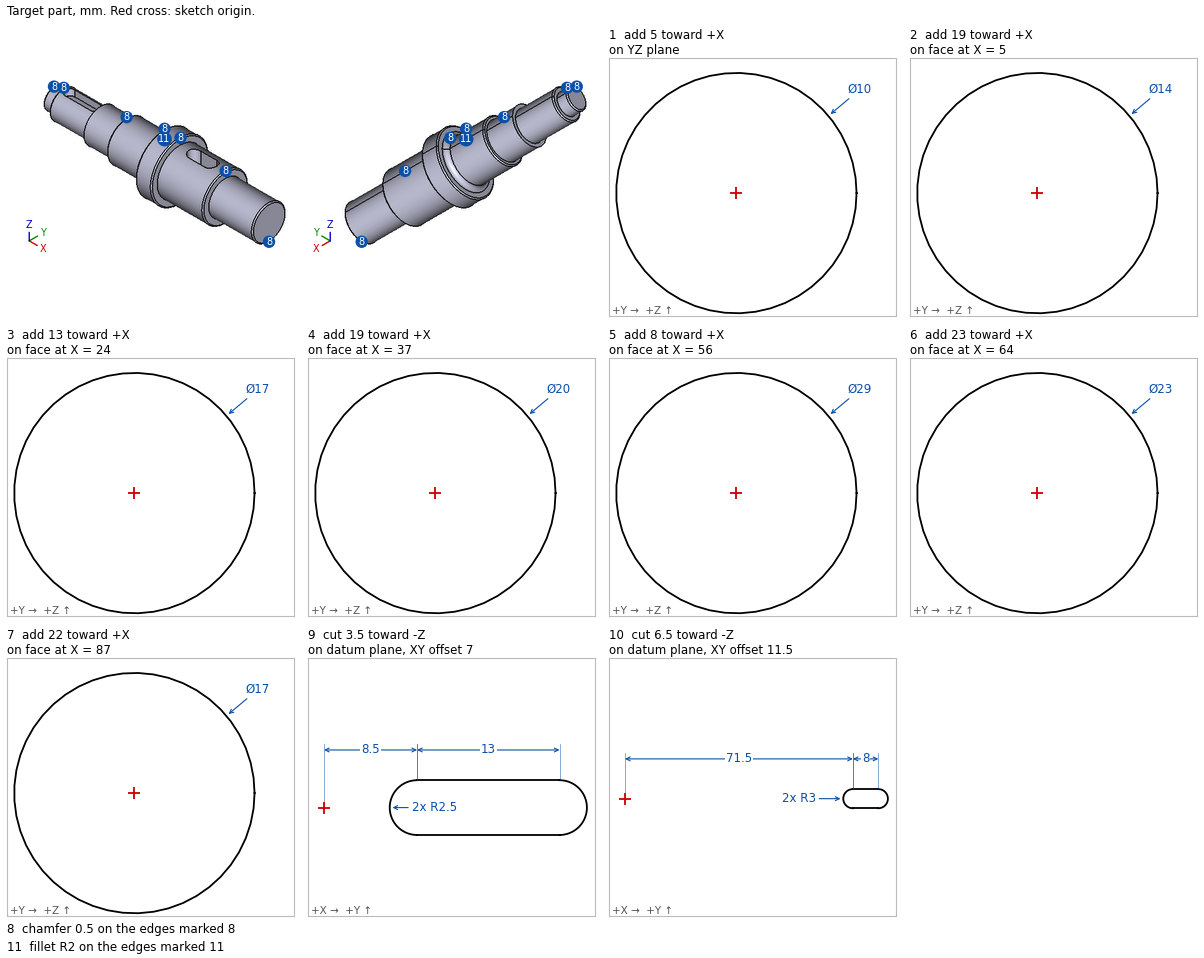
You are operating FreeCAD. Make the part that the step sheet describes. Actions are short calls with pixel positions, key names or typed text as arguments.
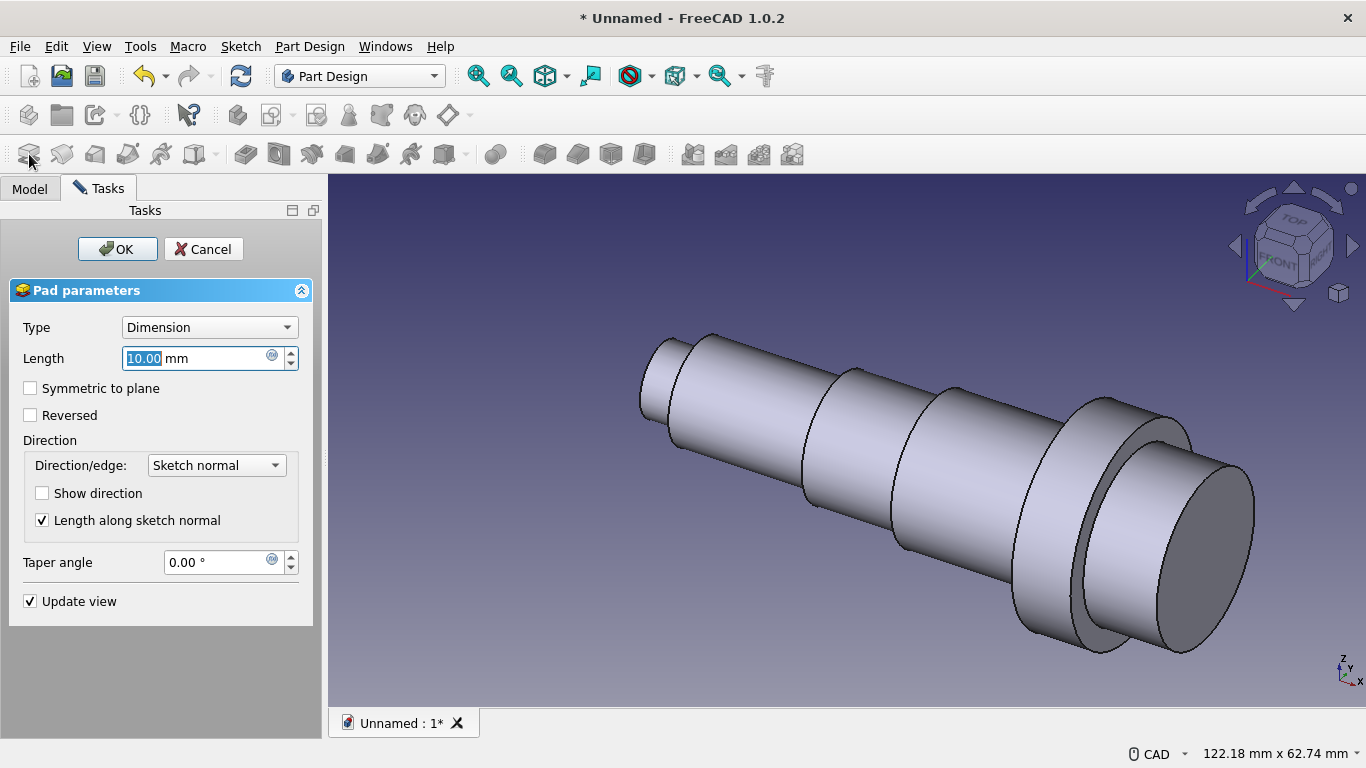
text(23)
key(Tab)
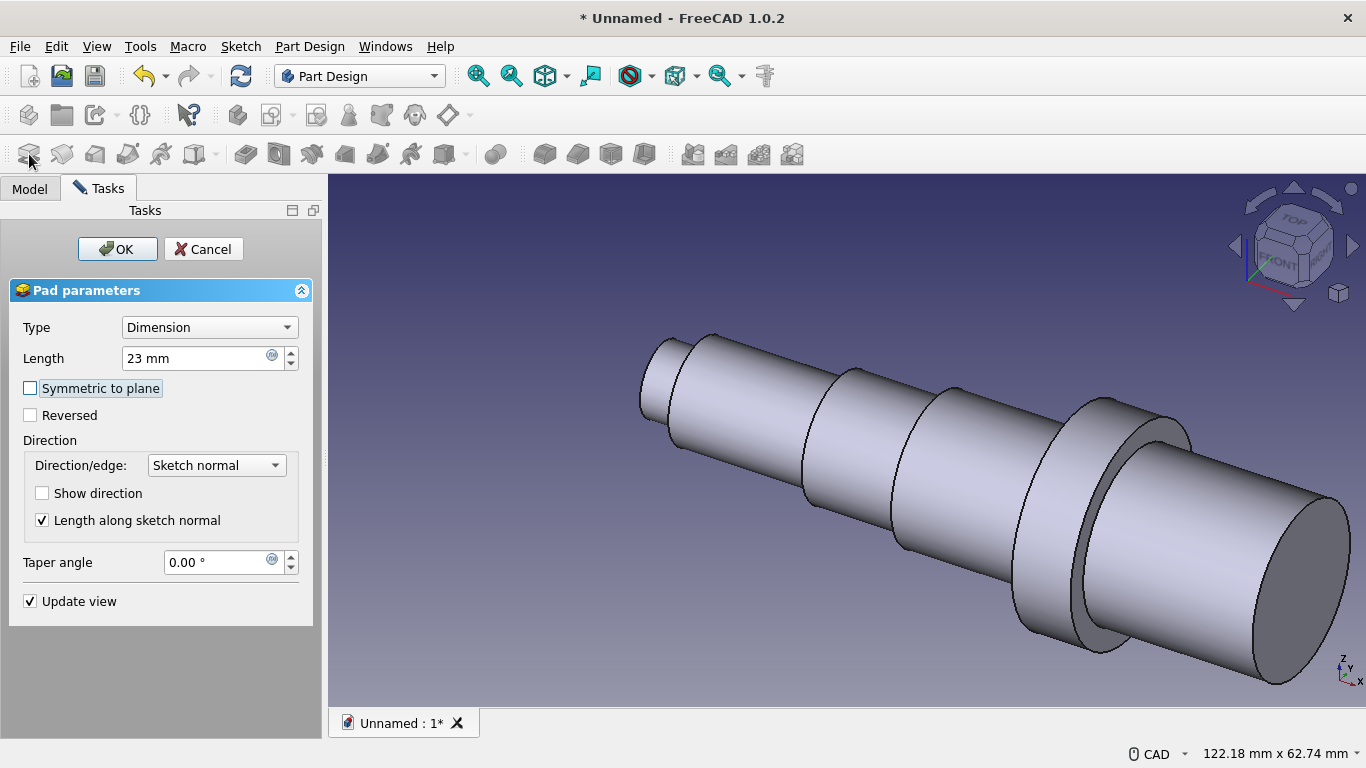
click(118, 249)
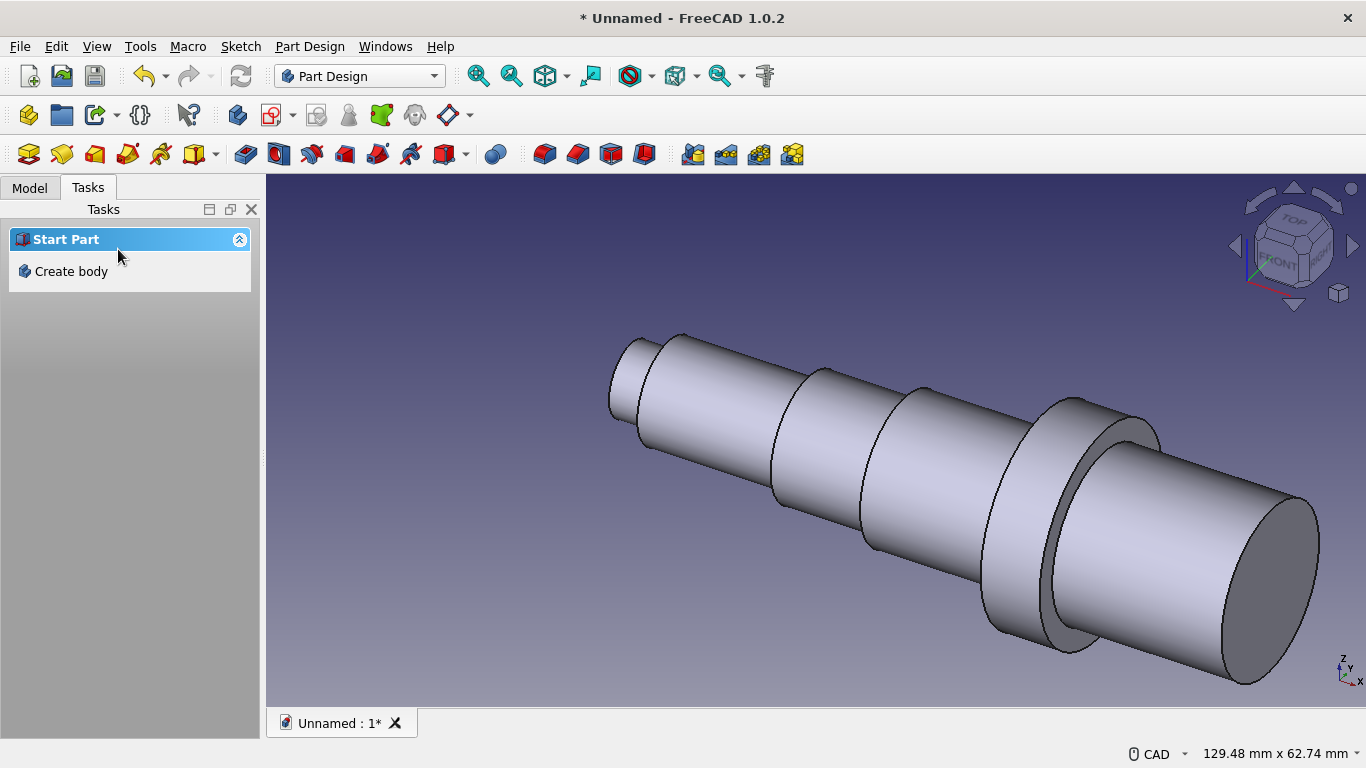
click(479, 76)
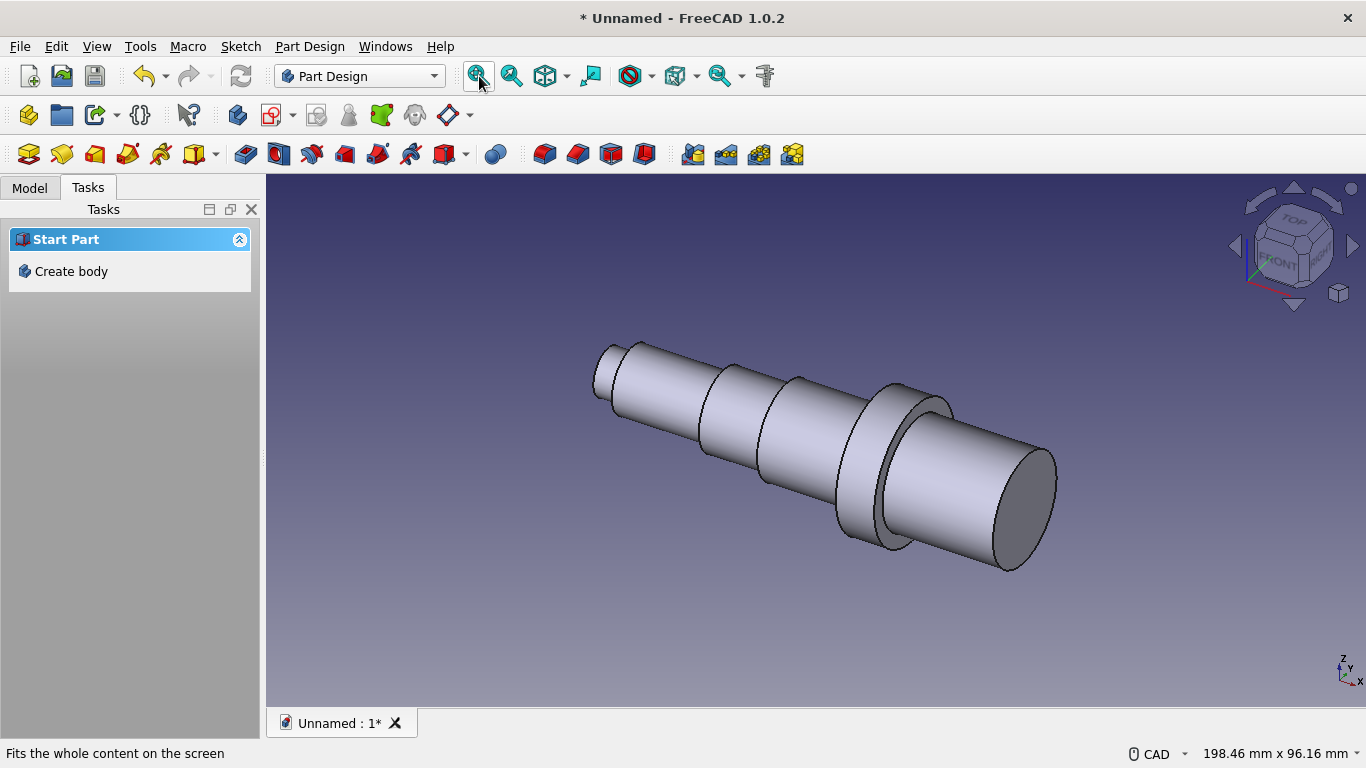
click(1025, 509)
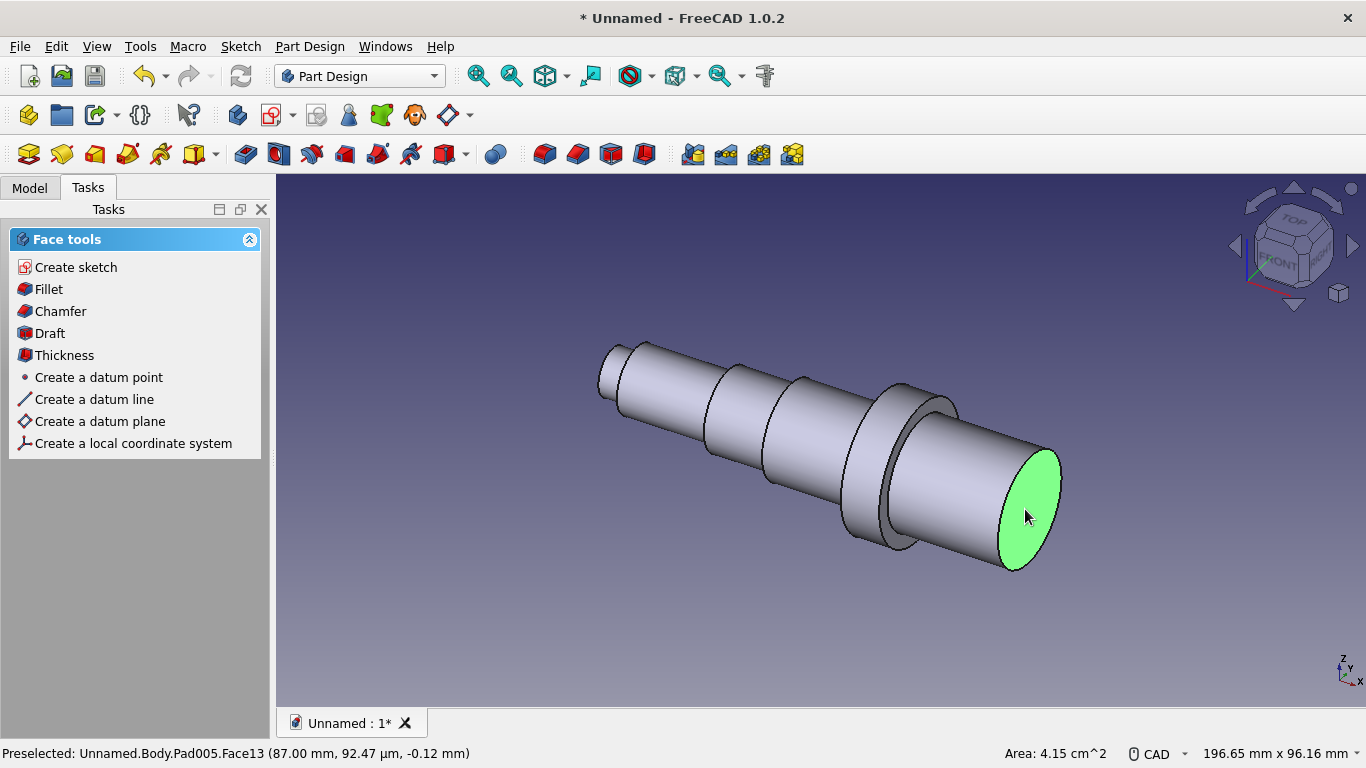
click(270, 116)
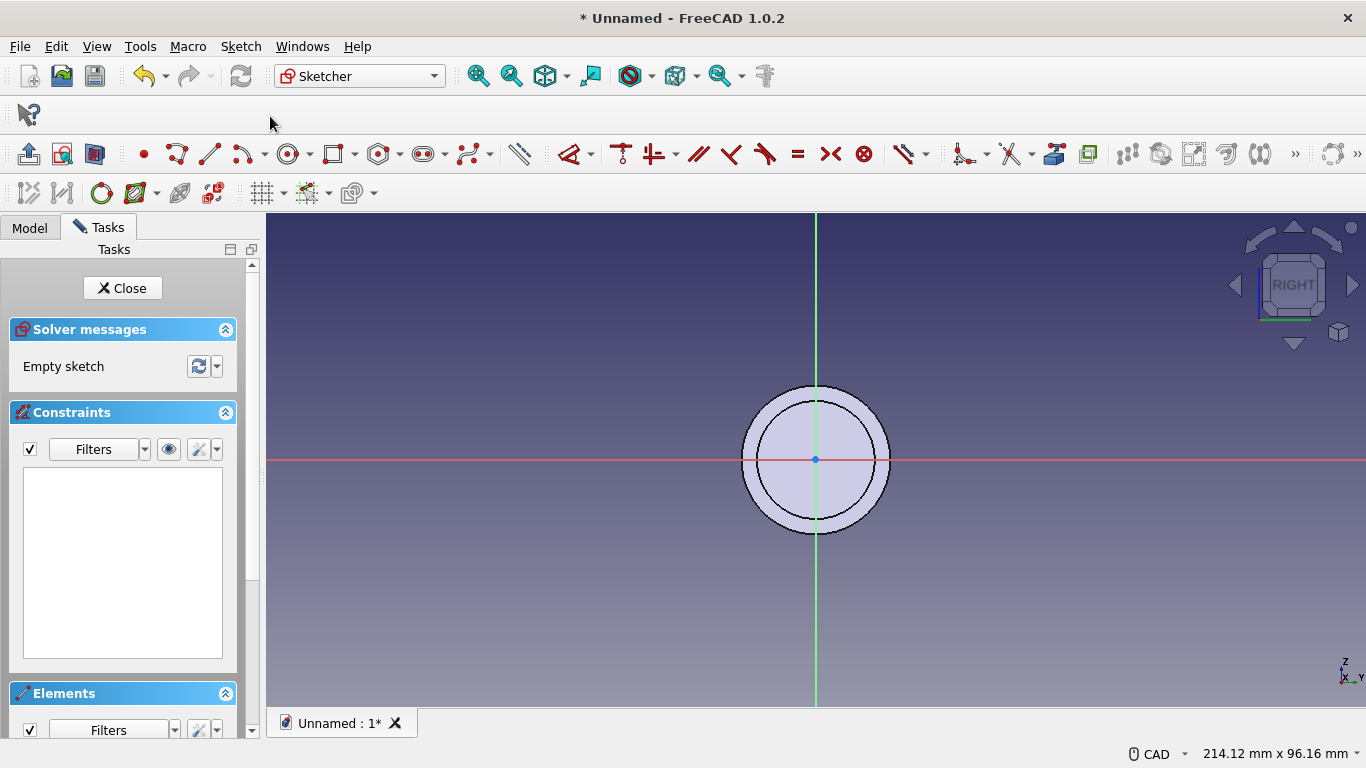
scroll(845, 460, up, 6)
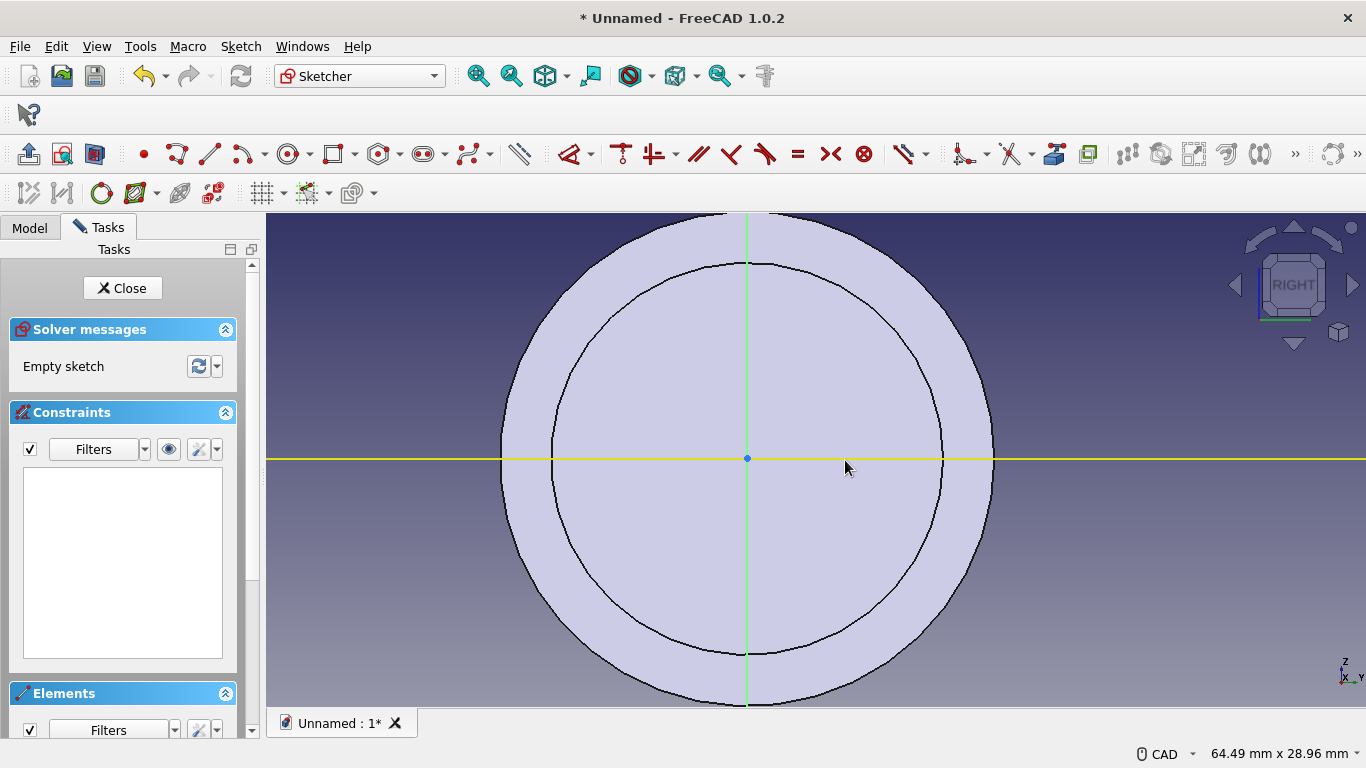
click(288, 154)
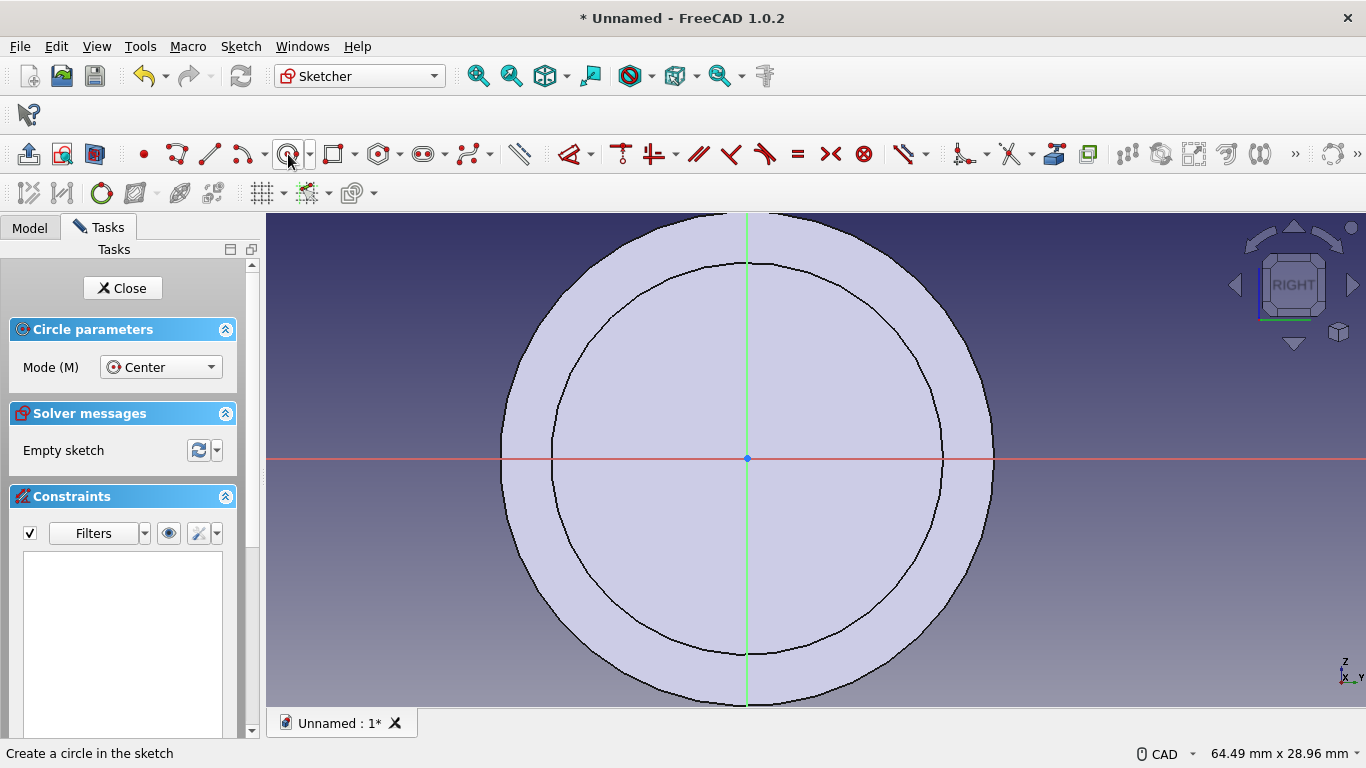
click(747, 459)
move(850, 356)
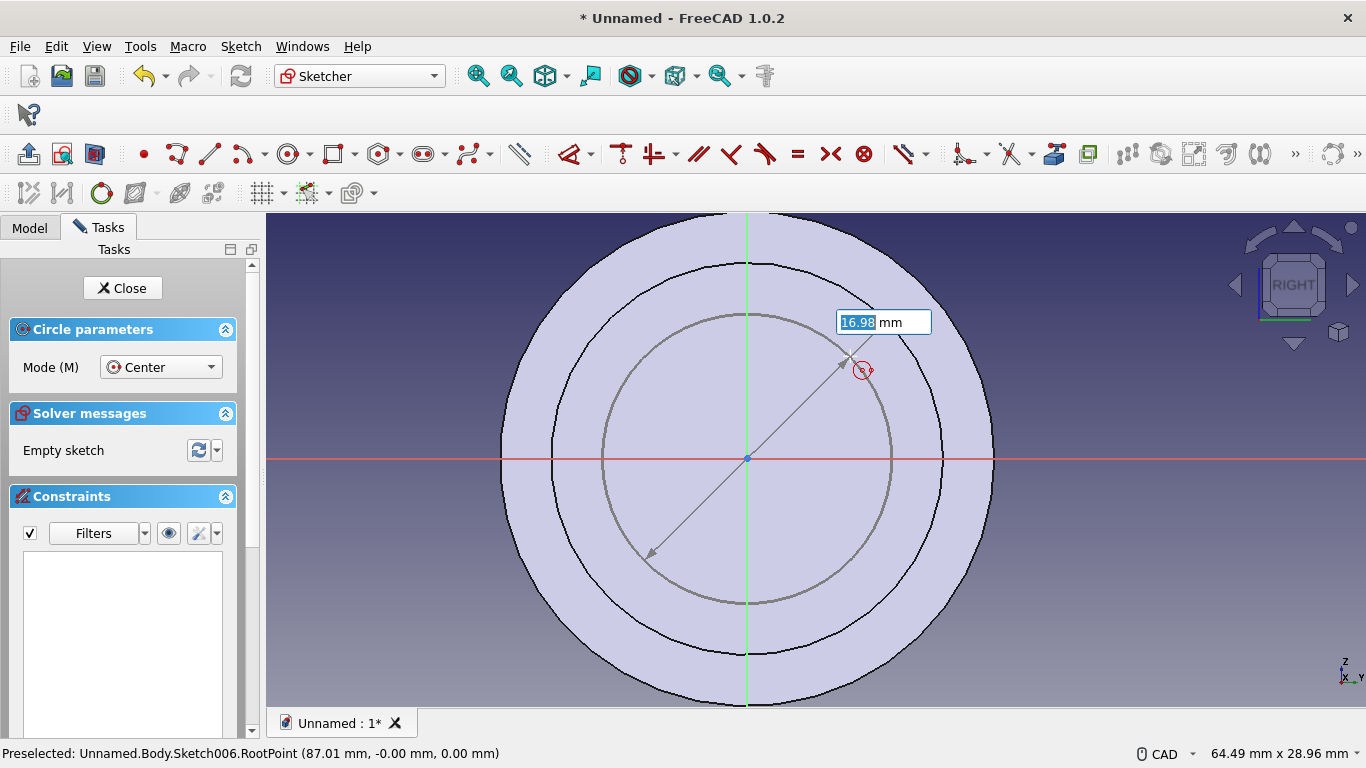
text(17)
key(Return)
key(Escape)